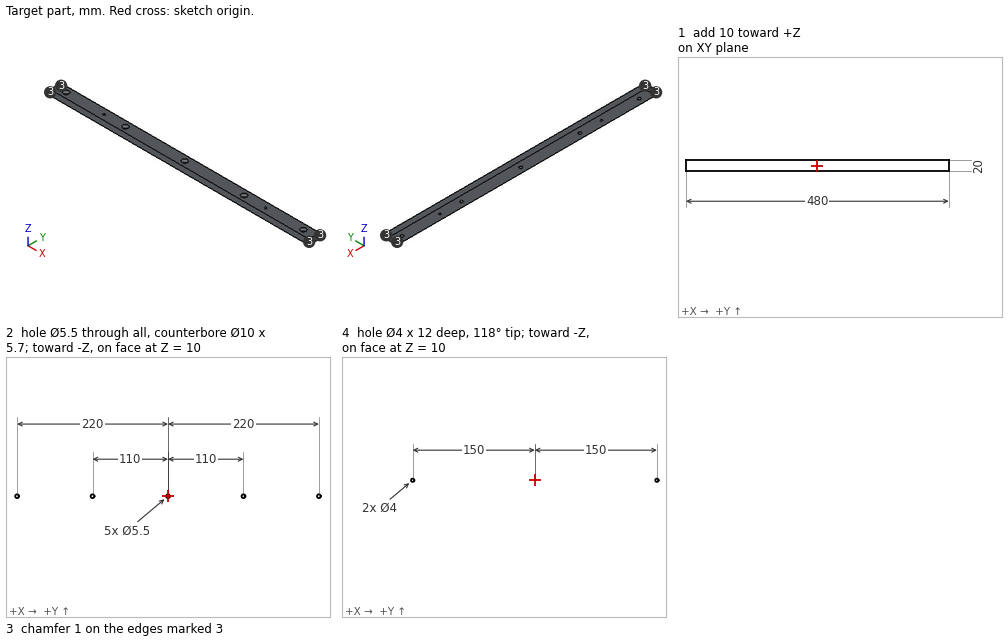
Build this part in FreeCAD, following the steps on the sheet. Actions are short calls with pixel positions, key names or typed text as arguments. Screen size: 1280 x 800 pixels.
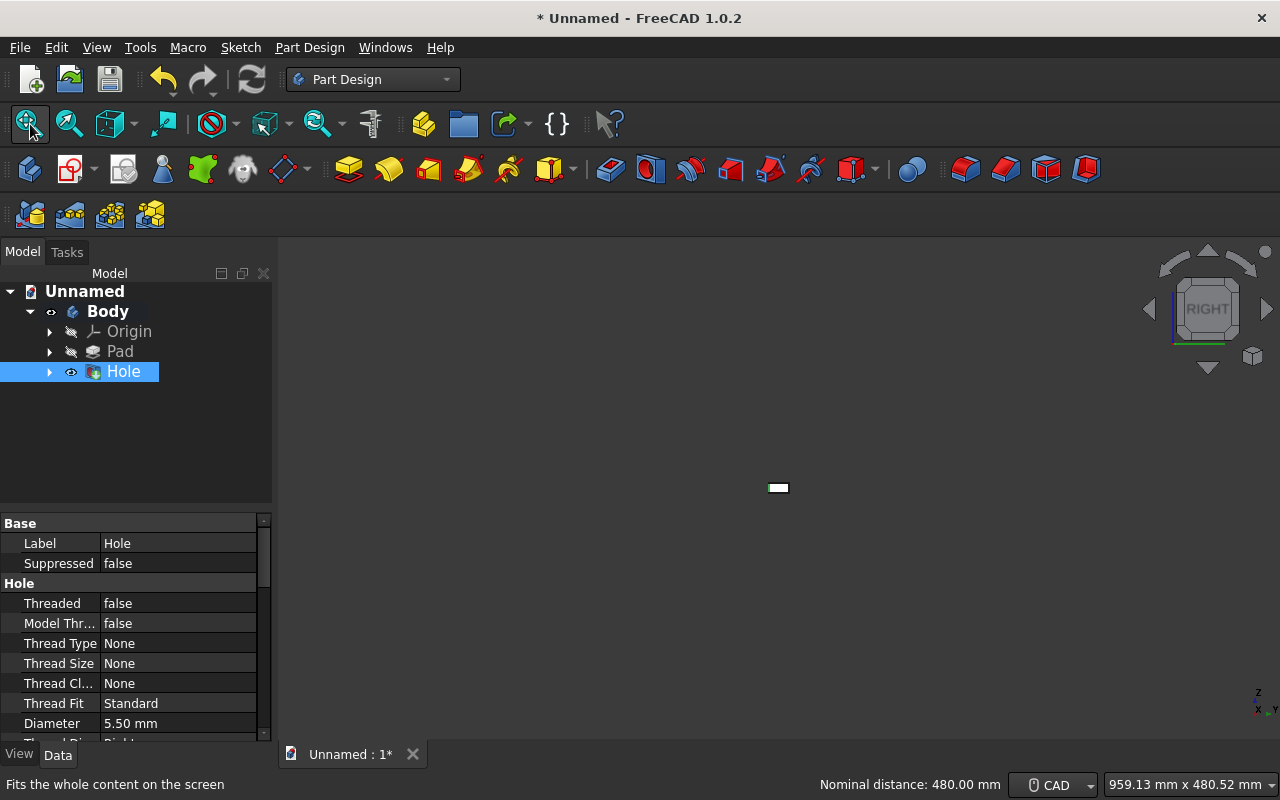
scroll(789, 487, up, 7)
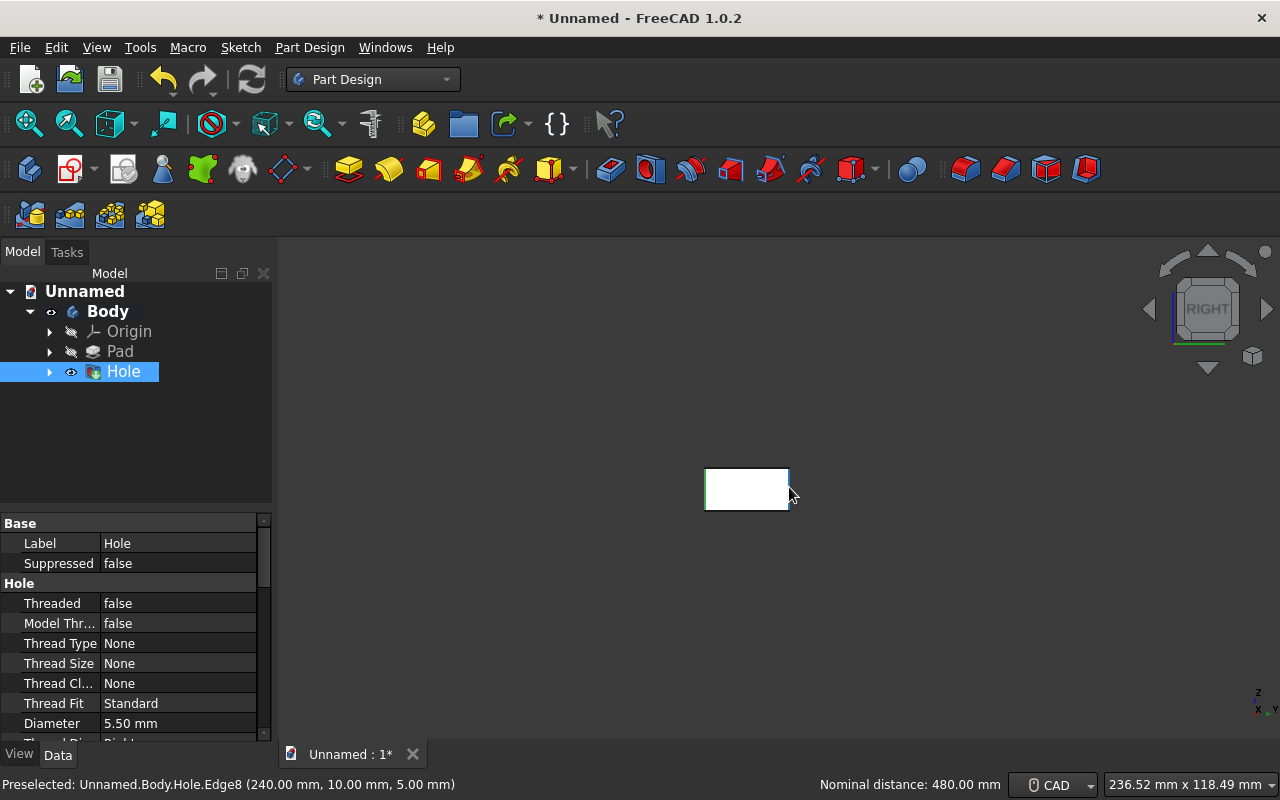
click(789, 489, ctrl)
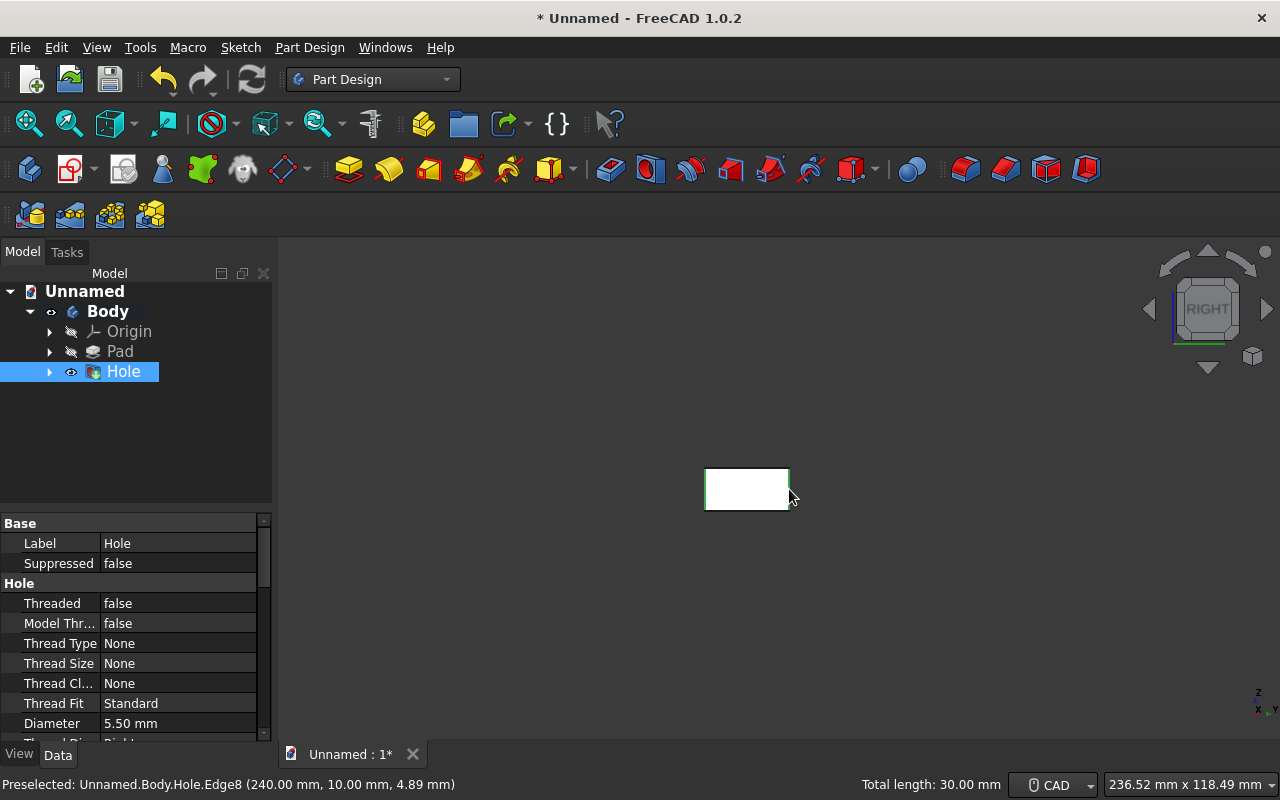
click(30, 124)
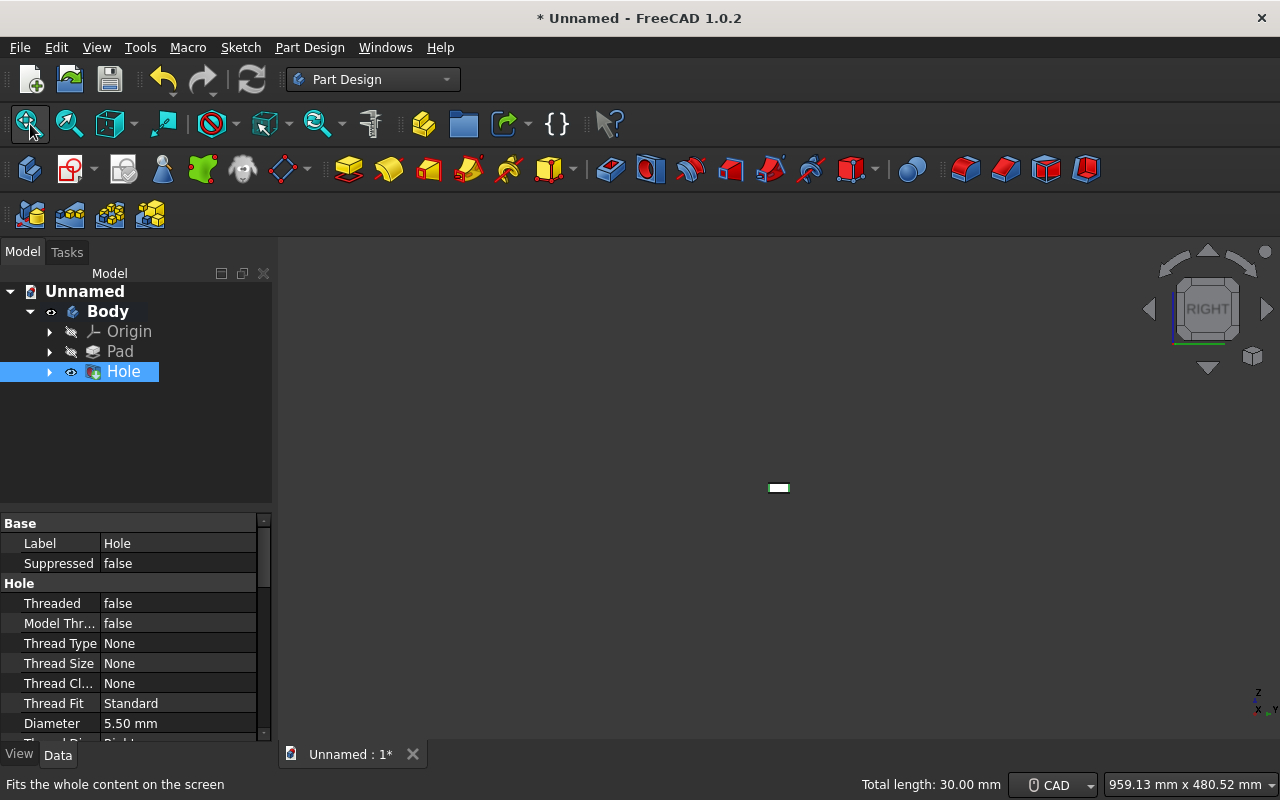
key(5)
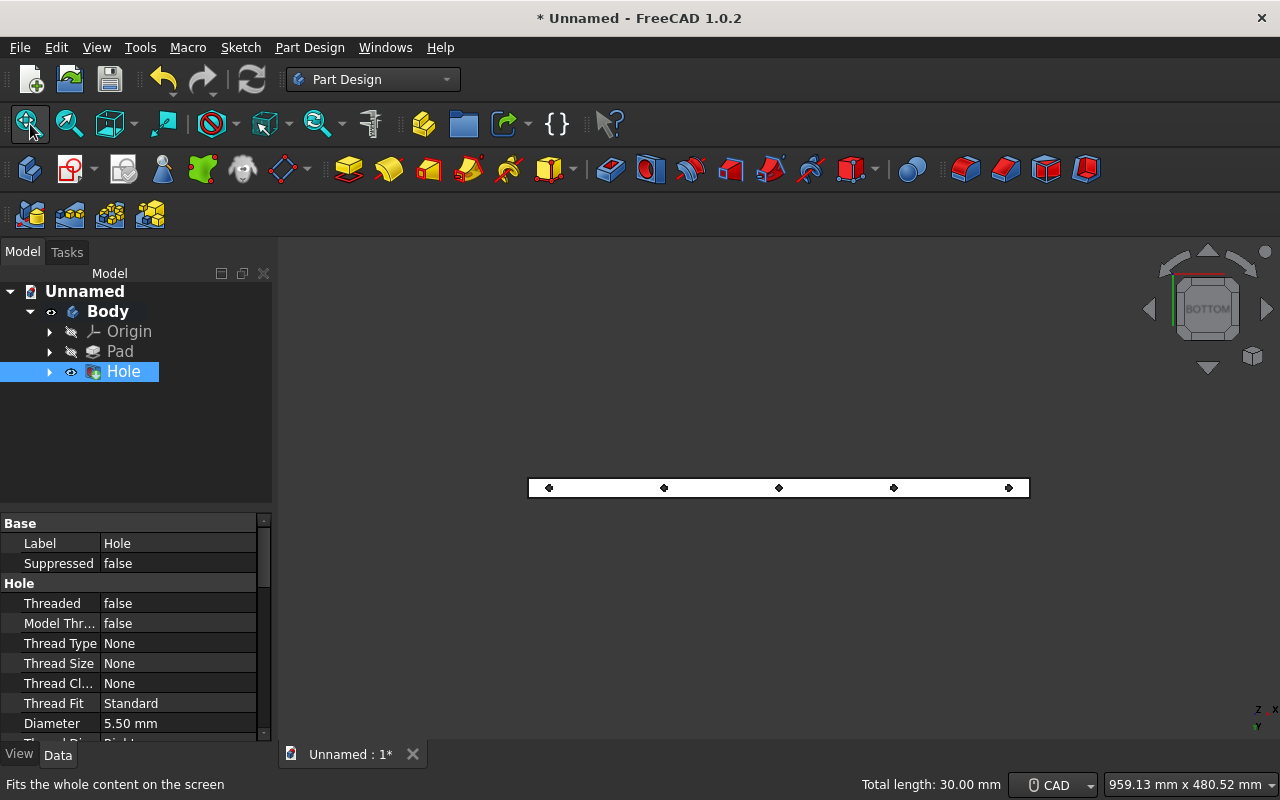
scroll(528, 497, up, 7)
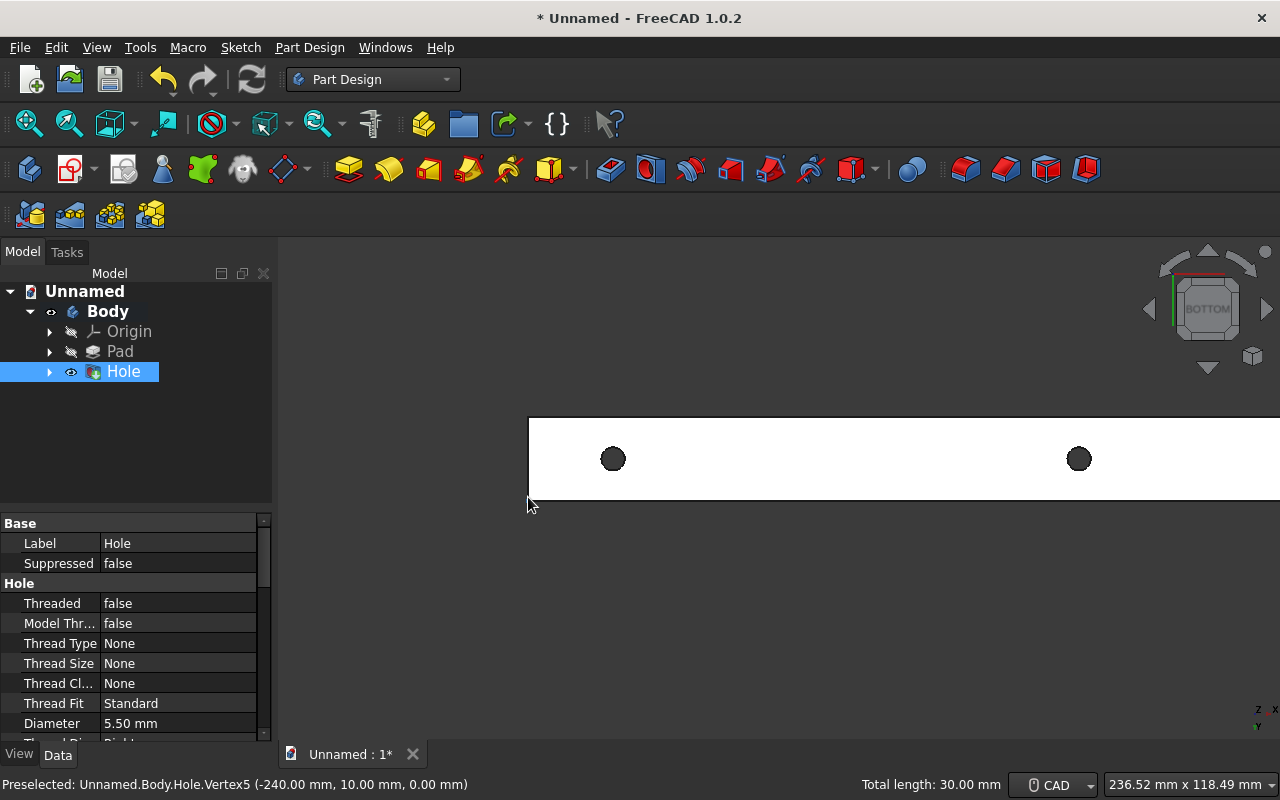
click(30, 124)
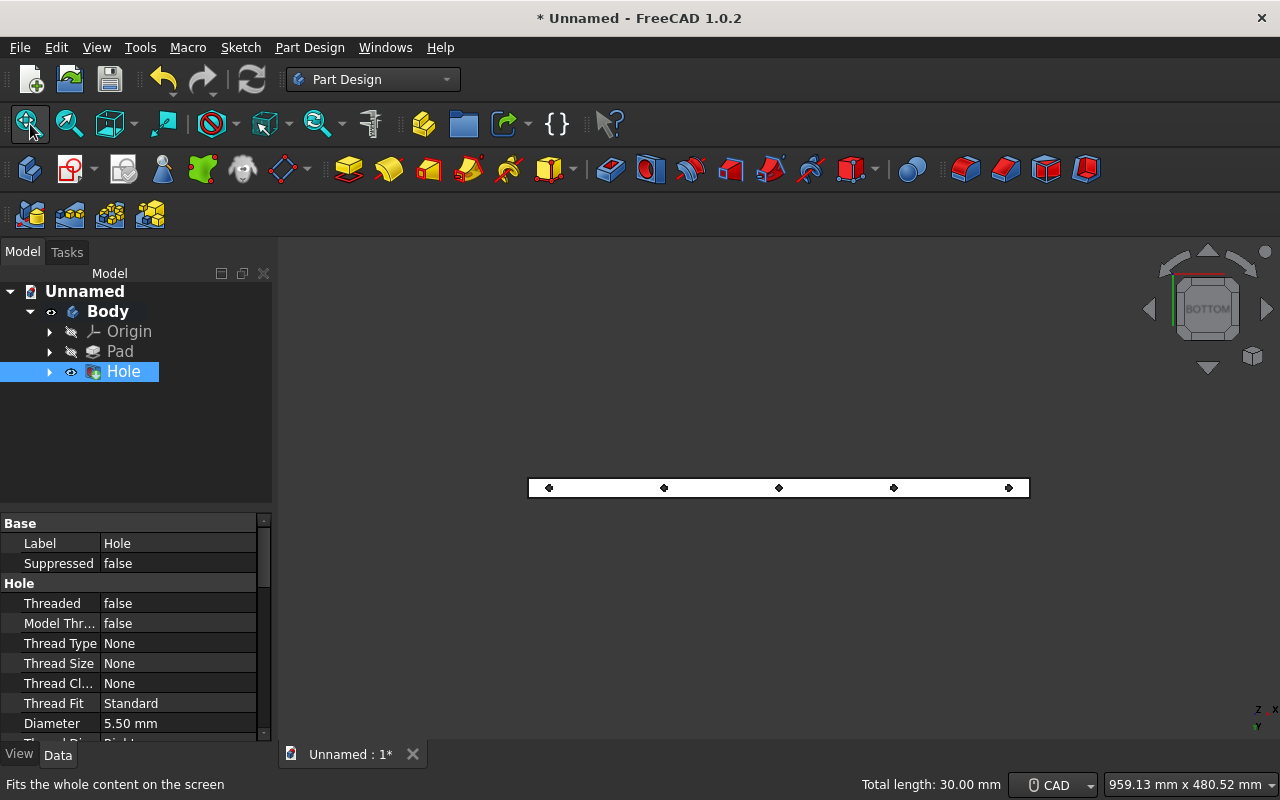
key(4)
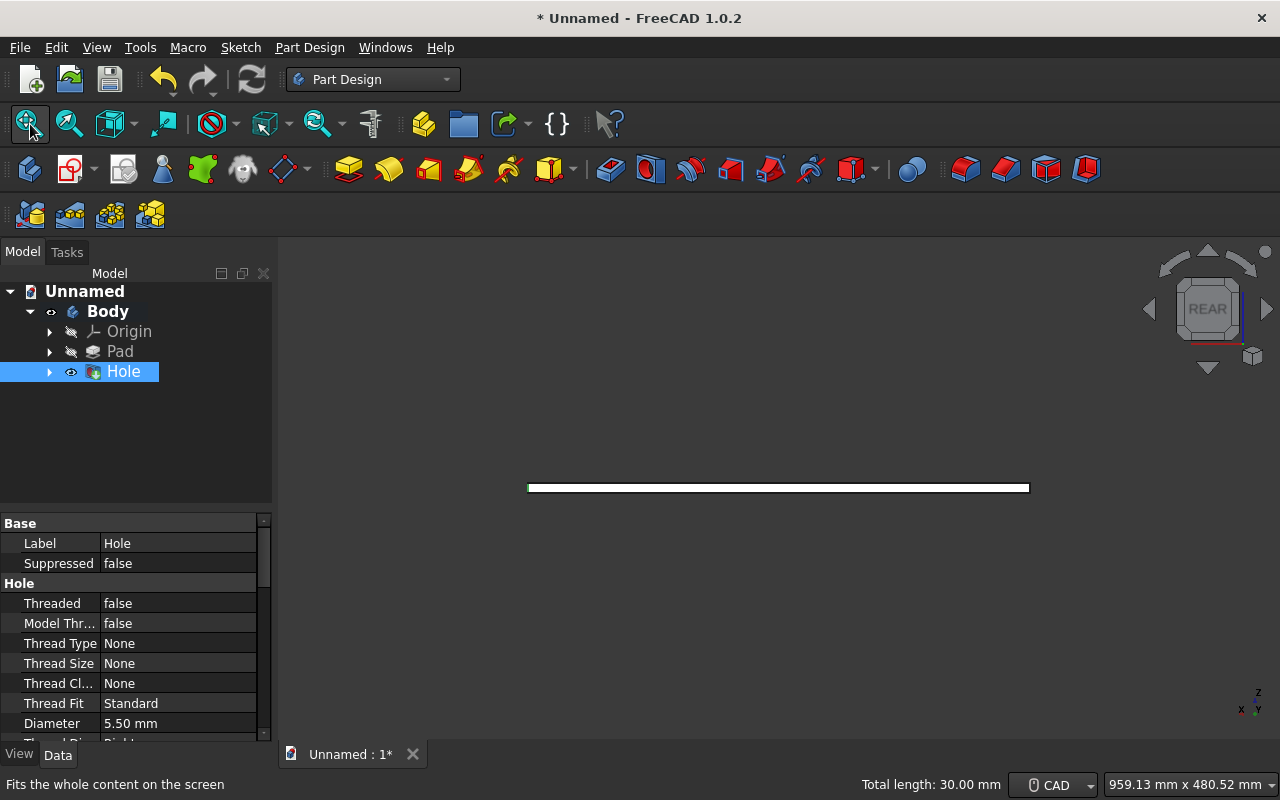
scroll(1030, 487, up, 7)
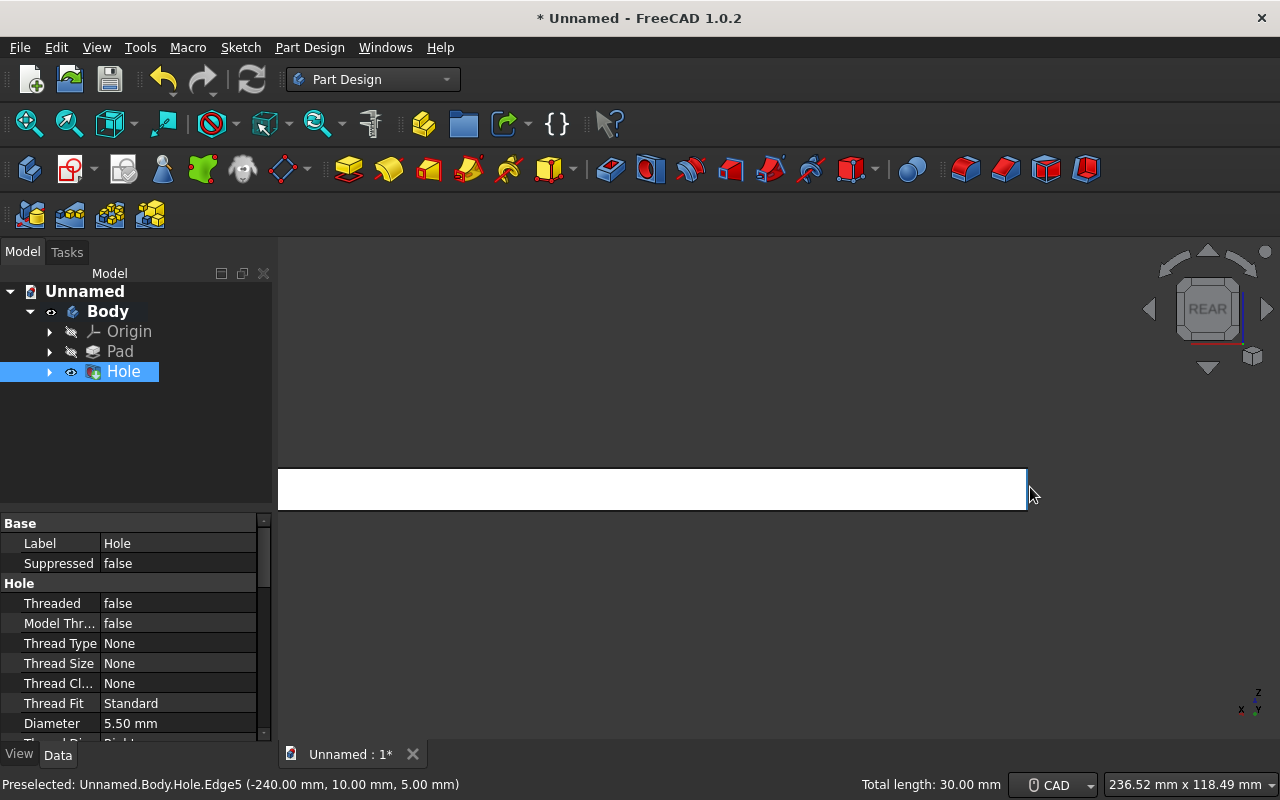
click(1027, 489, ctrl)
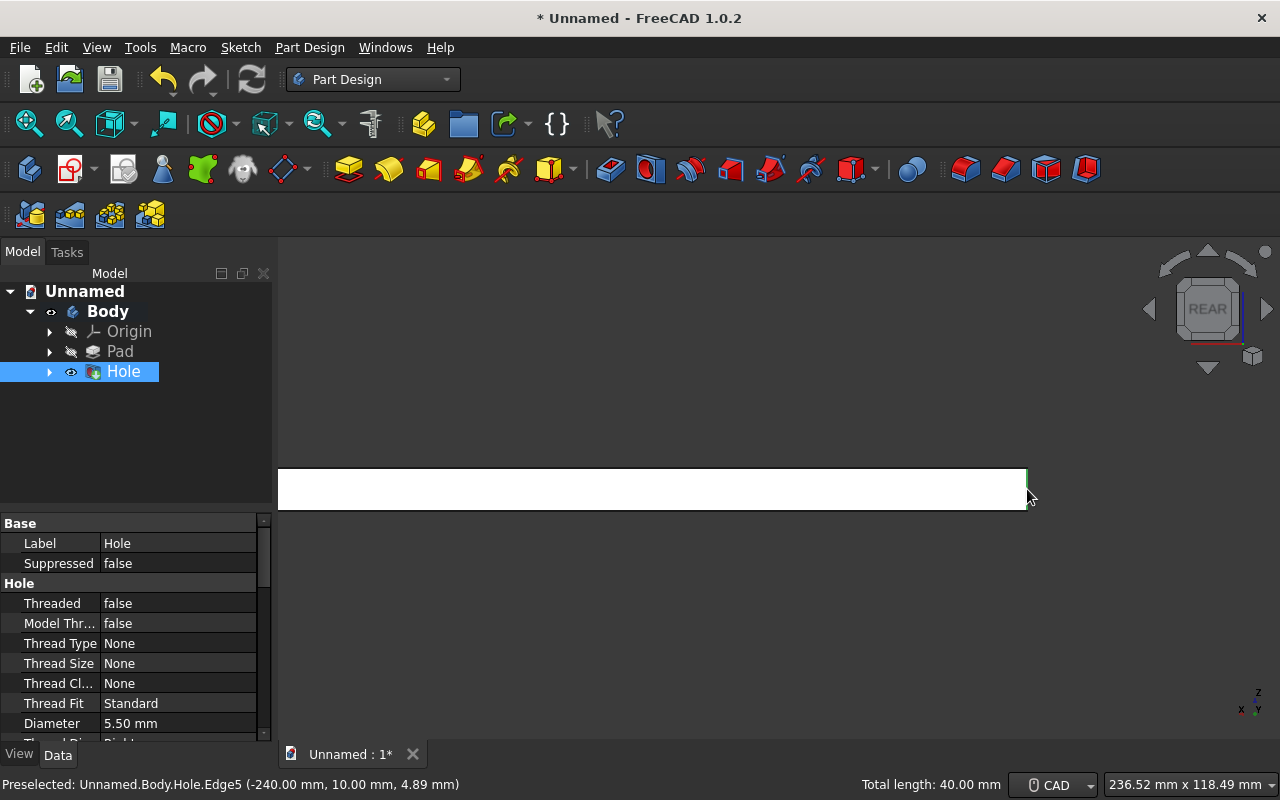
click(1006, 170)